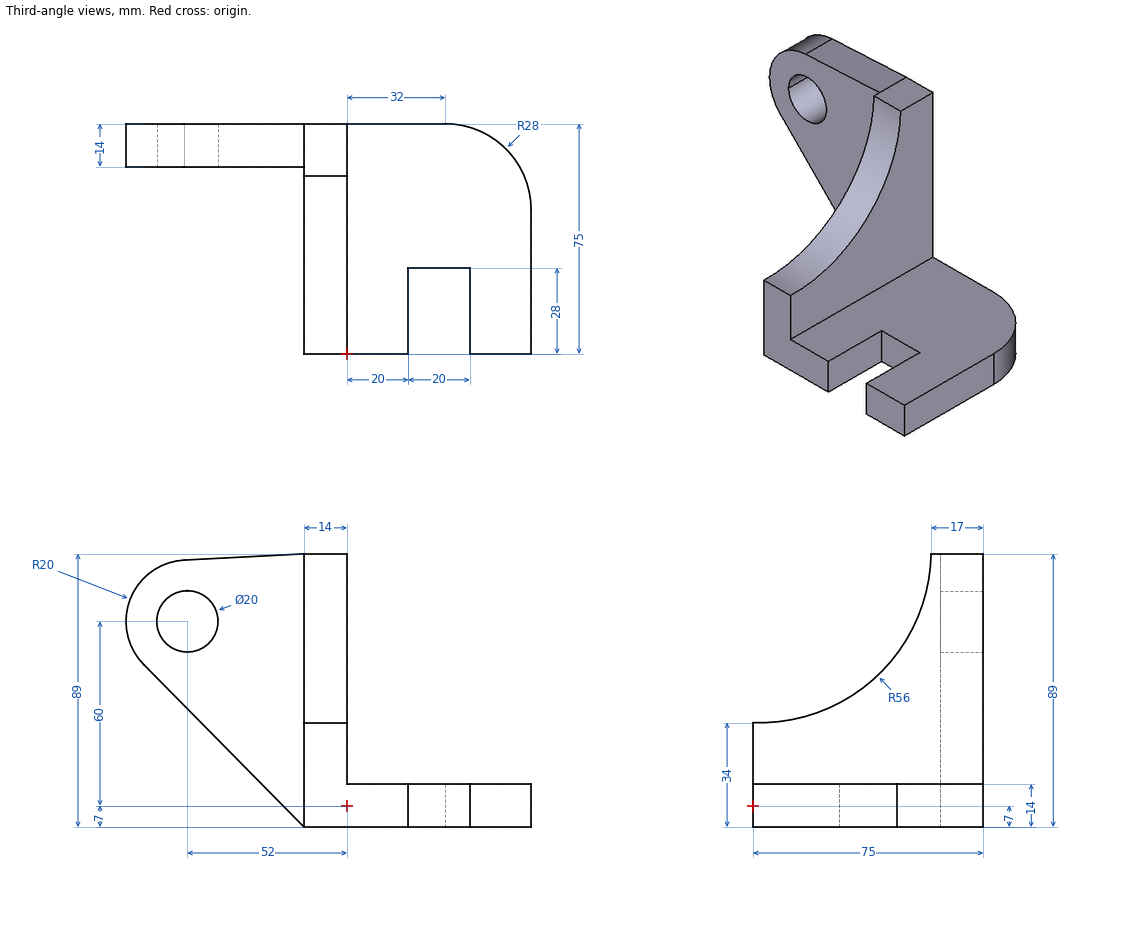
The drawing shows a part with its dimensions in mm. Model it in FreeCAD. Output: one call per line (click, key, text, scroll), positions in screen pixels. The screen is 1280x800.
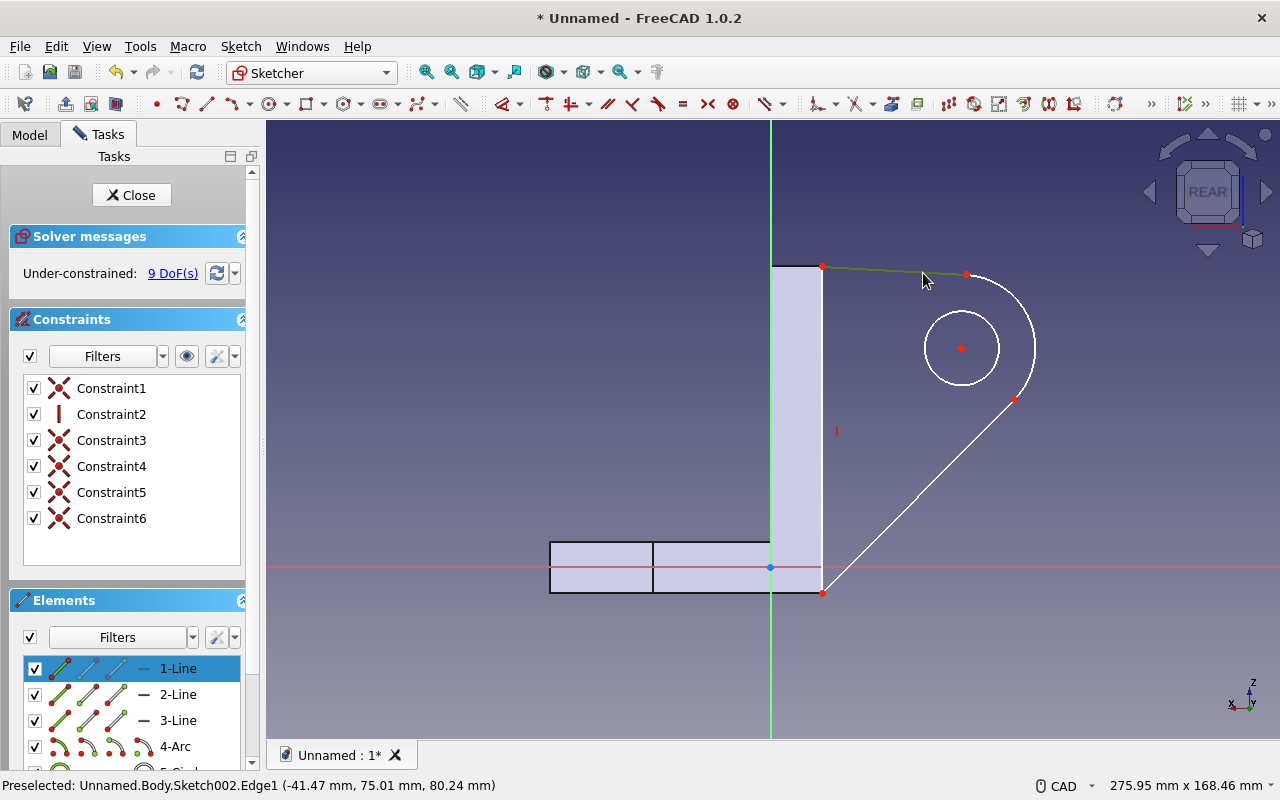
click(1035, 355)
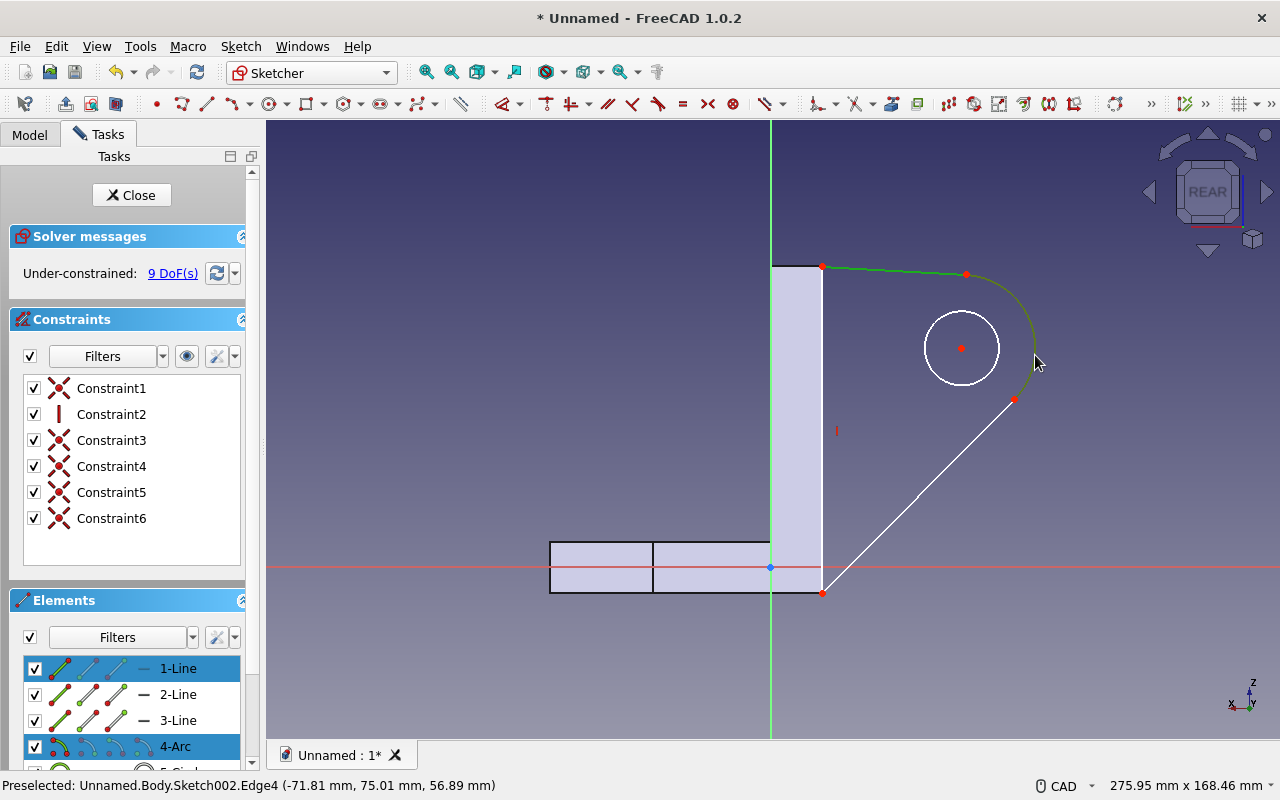
click(658, 104)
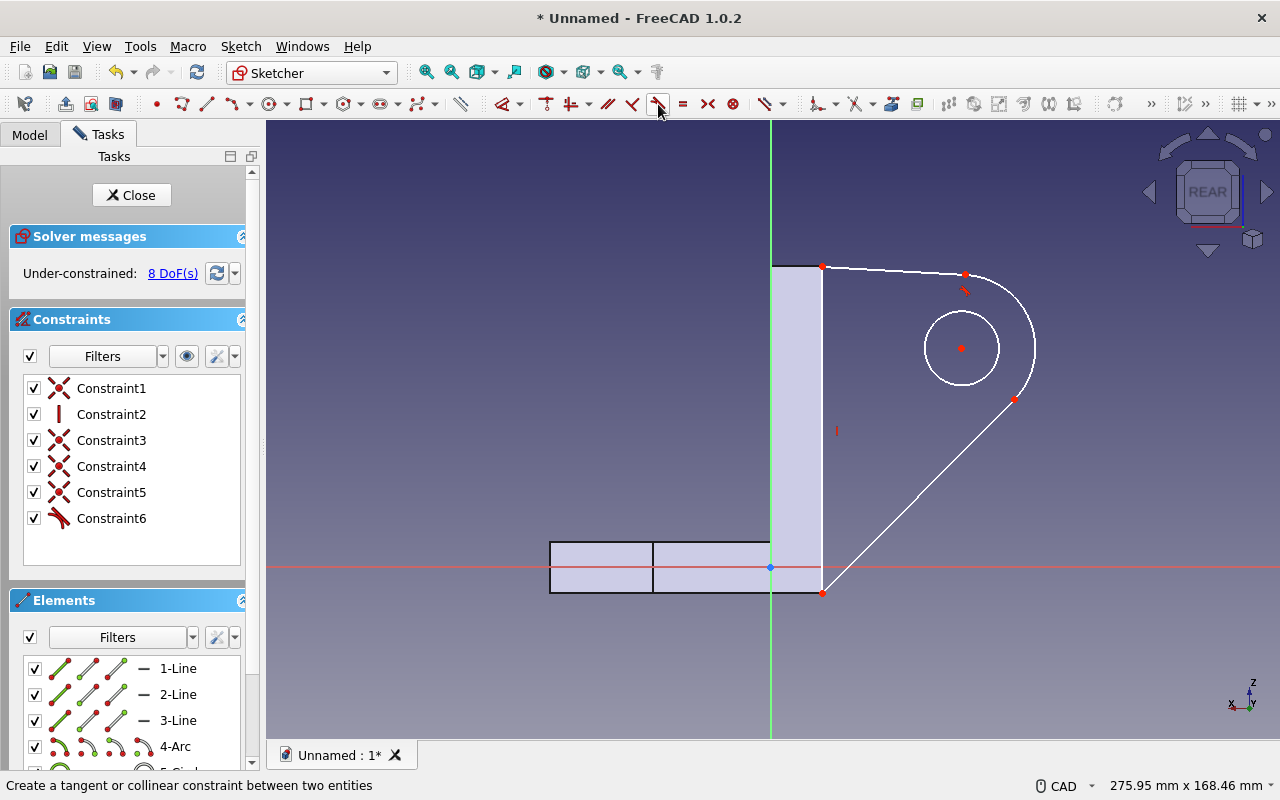
click(880, 536)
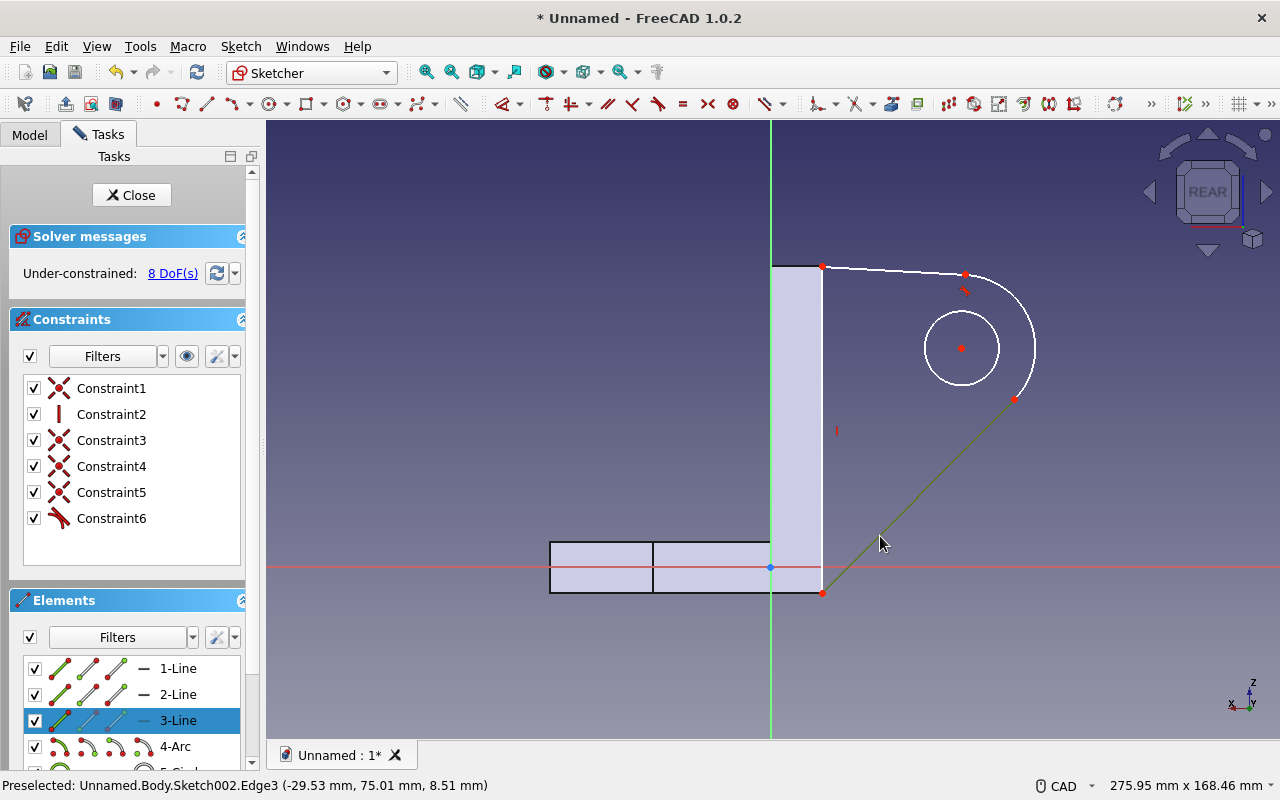
click(1035, 355)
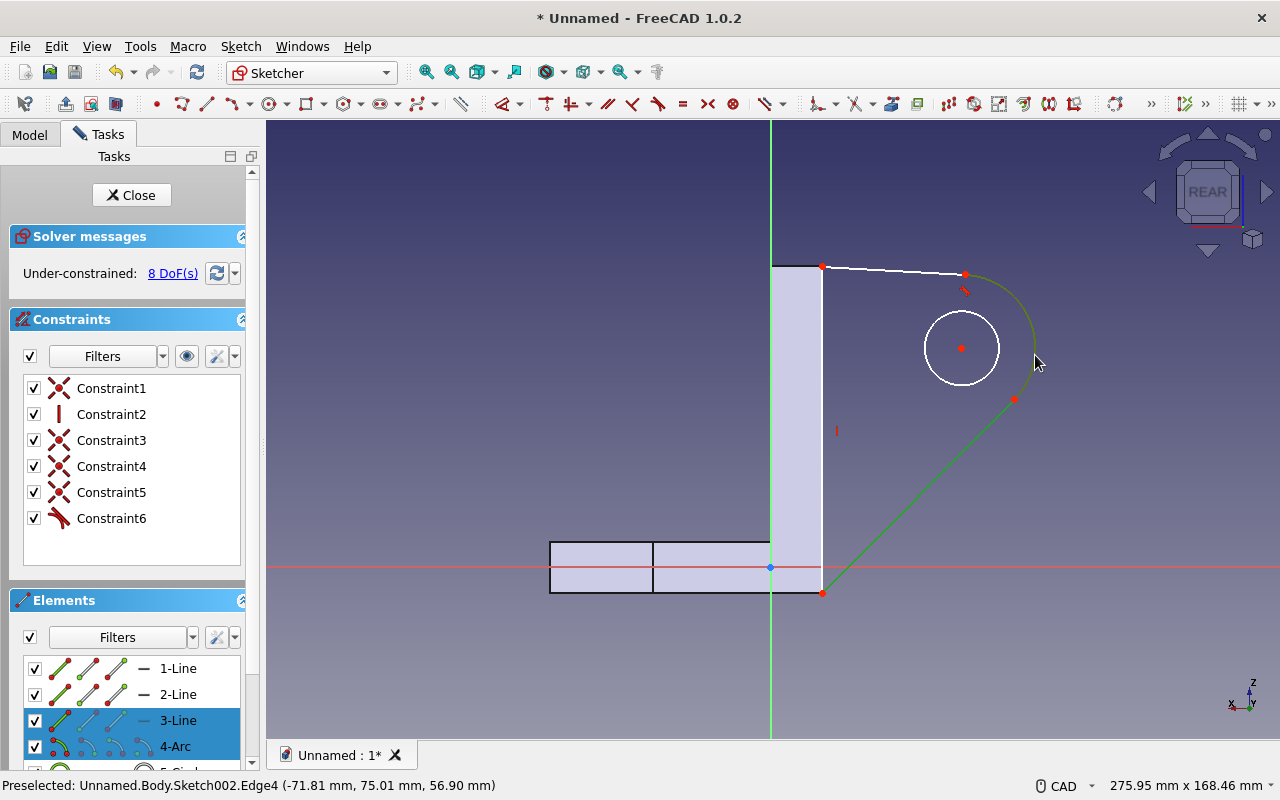
click(658, 104)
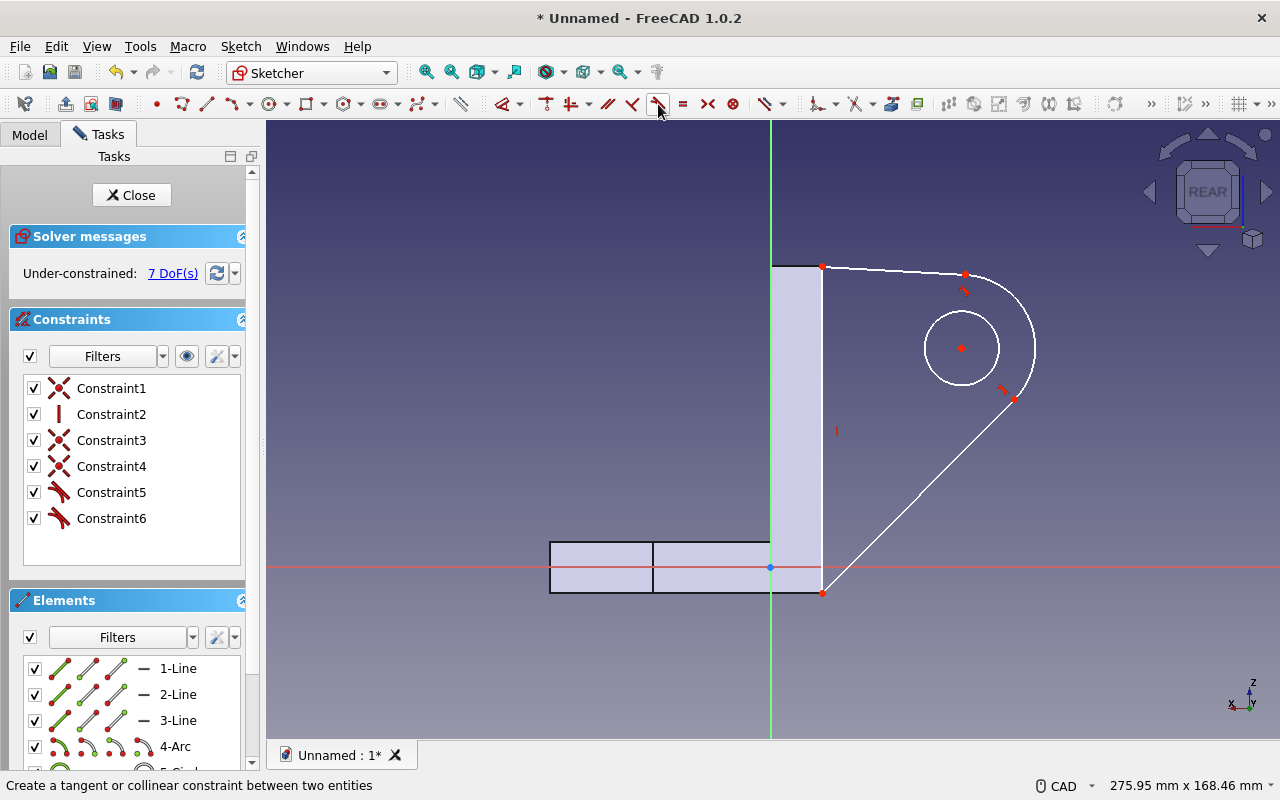
click(502, 104)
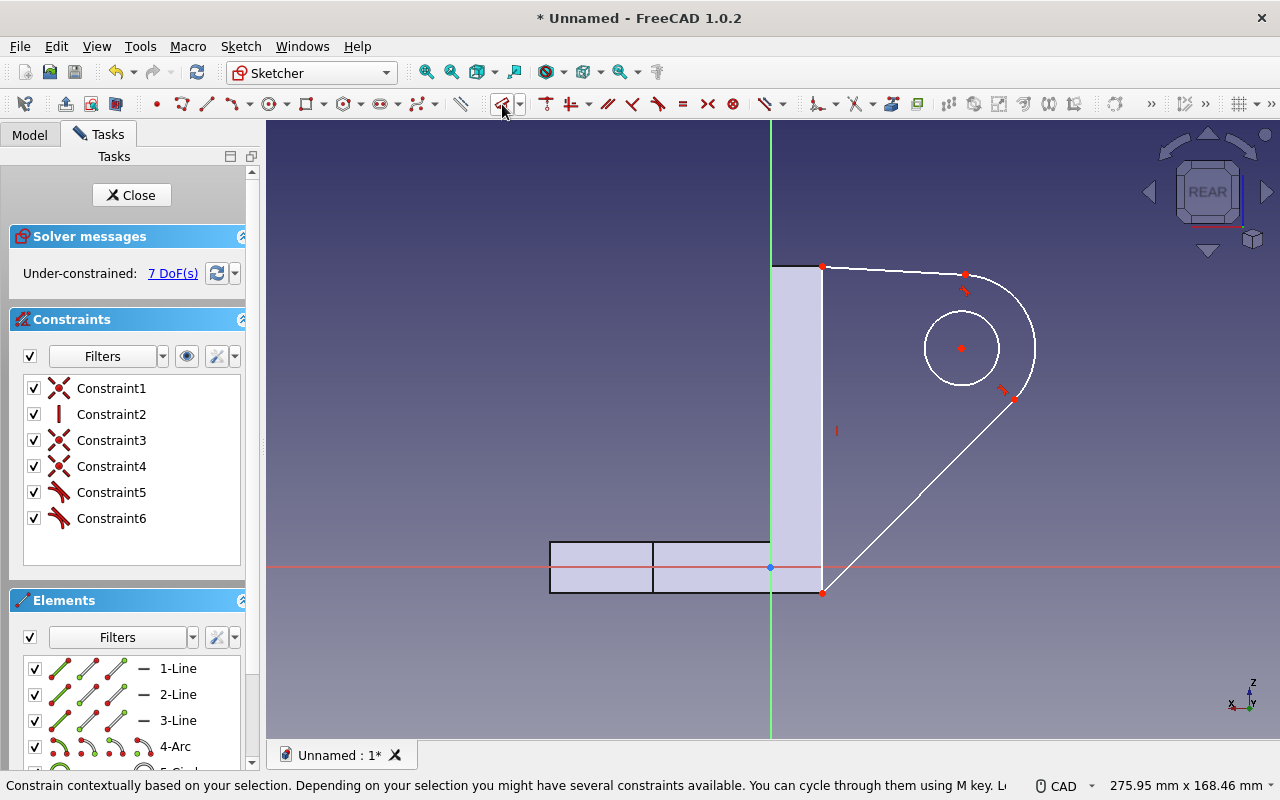
click(1035, 355)
click(1067, 358)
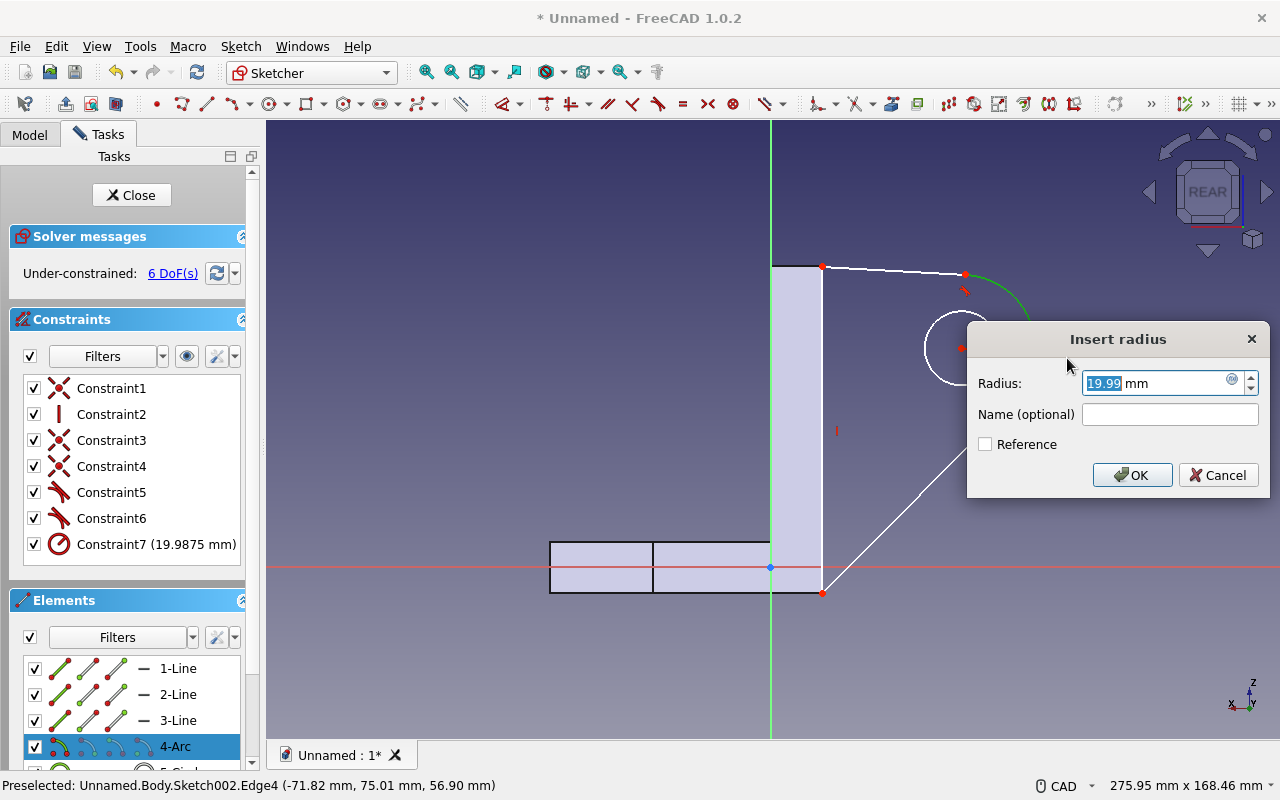
text(20)
key(Return)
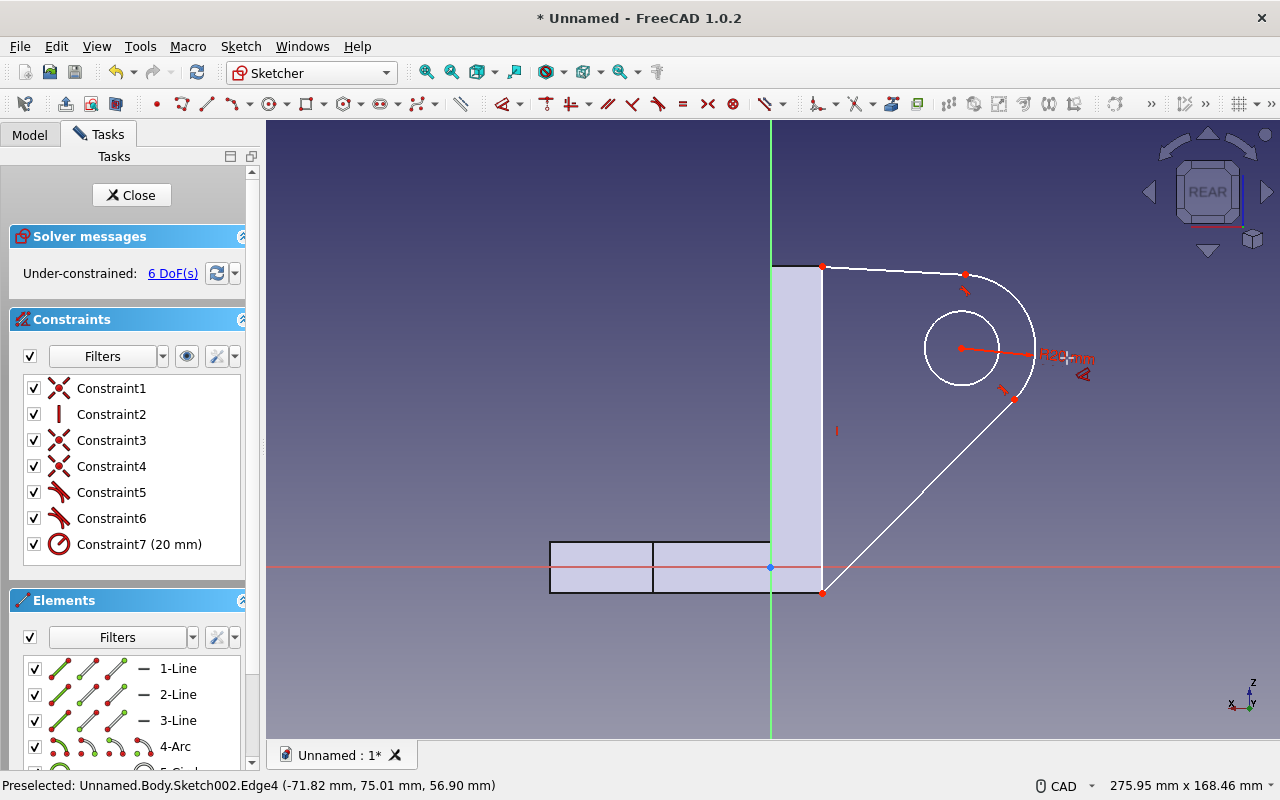
click(988, 322)
click(913, 300)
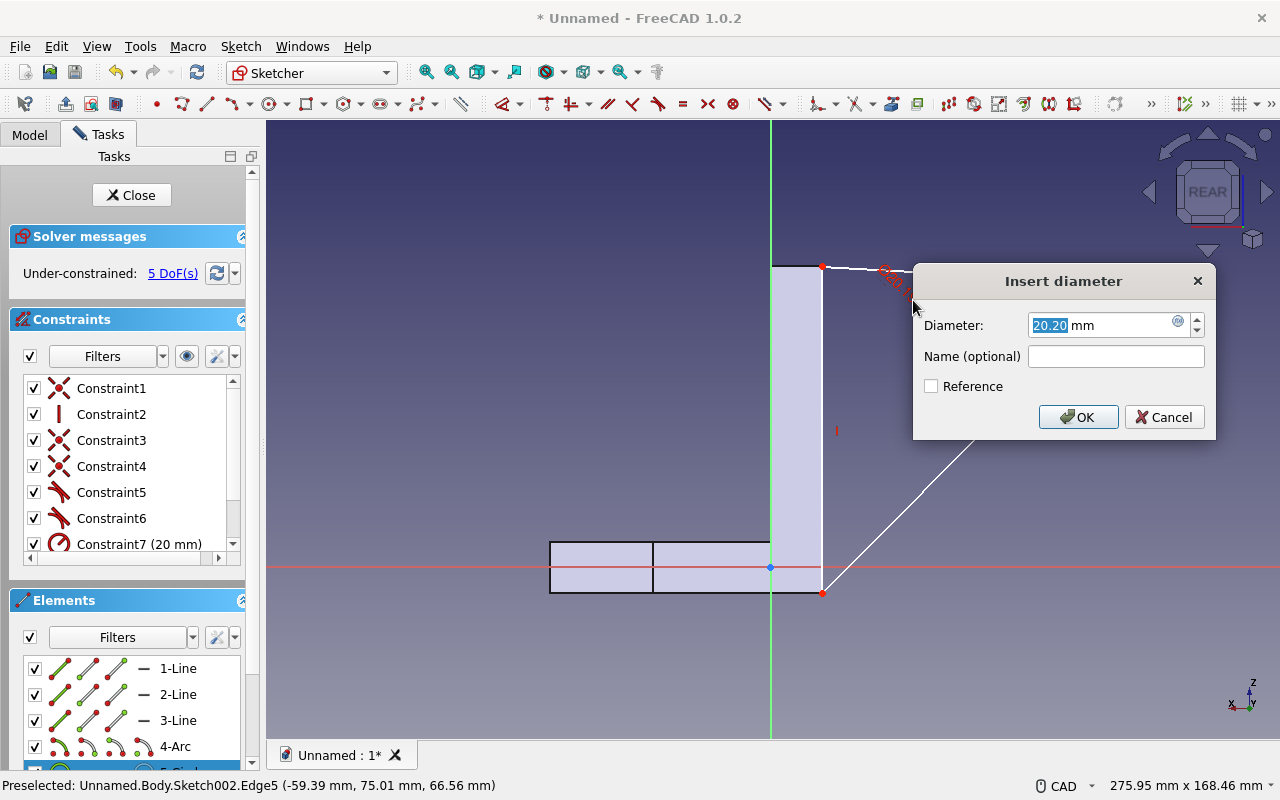
text(20)
key(Return)